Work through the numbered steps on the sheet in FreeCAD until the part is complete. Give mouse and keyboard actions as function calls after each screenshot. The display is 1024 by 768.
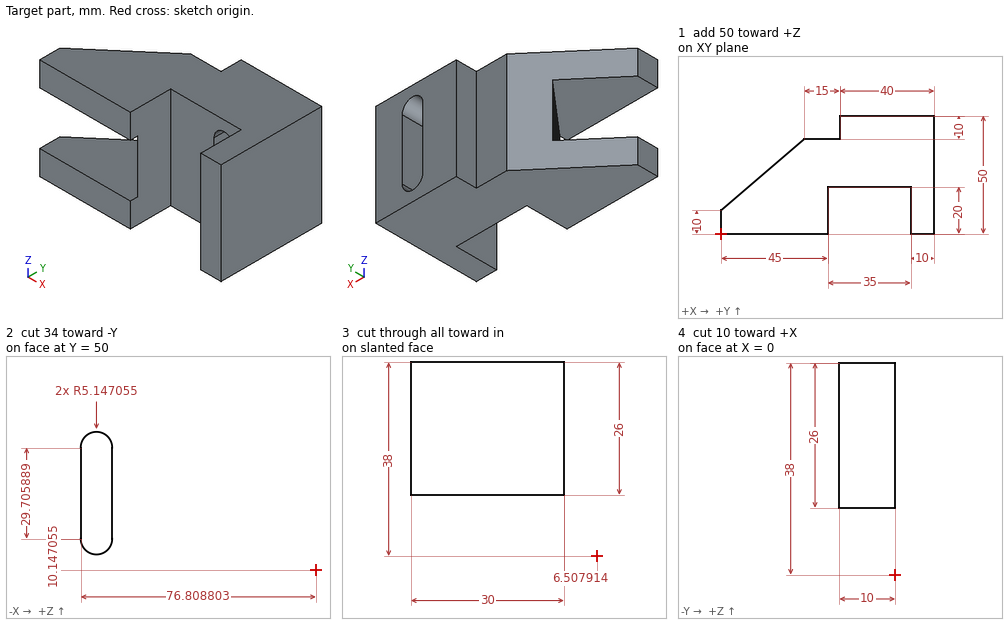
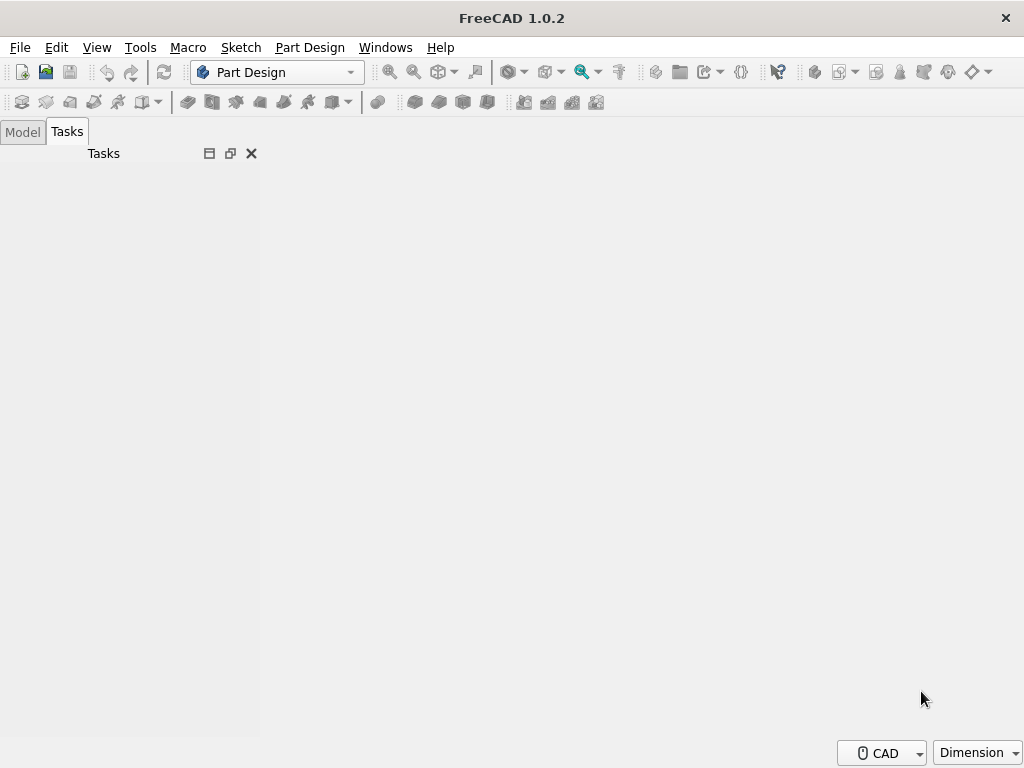
key(ctrl+n)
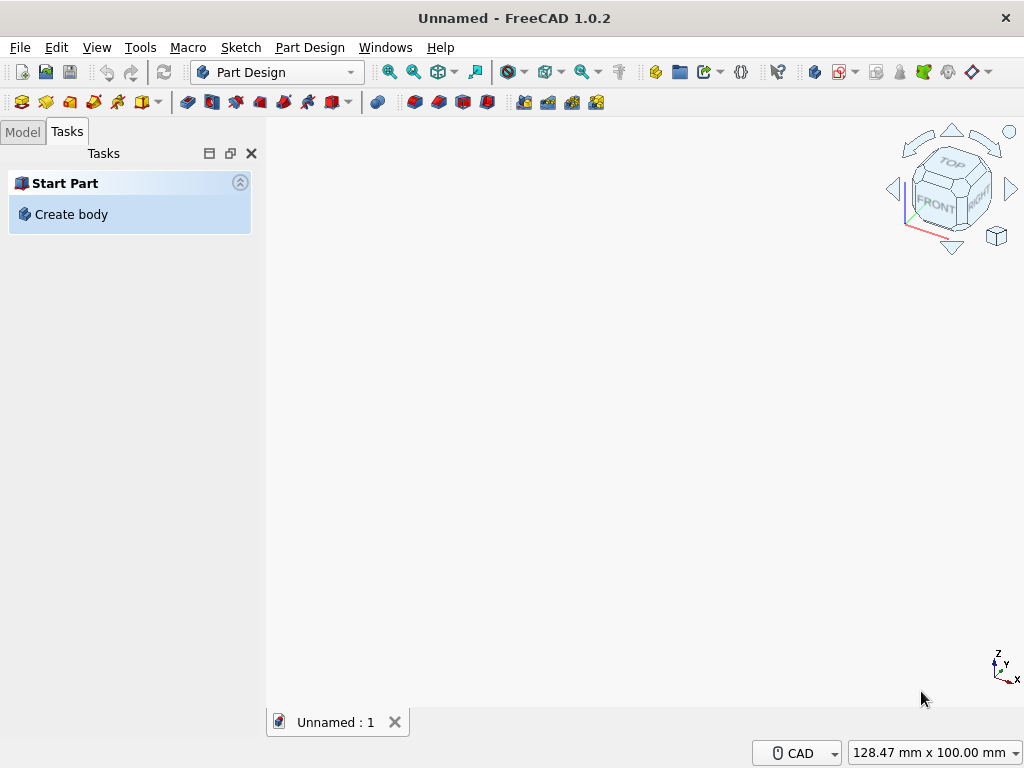
click(840, 72)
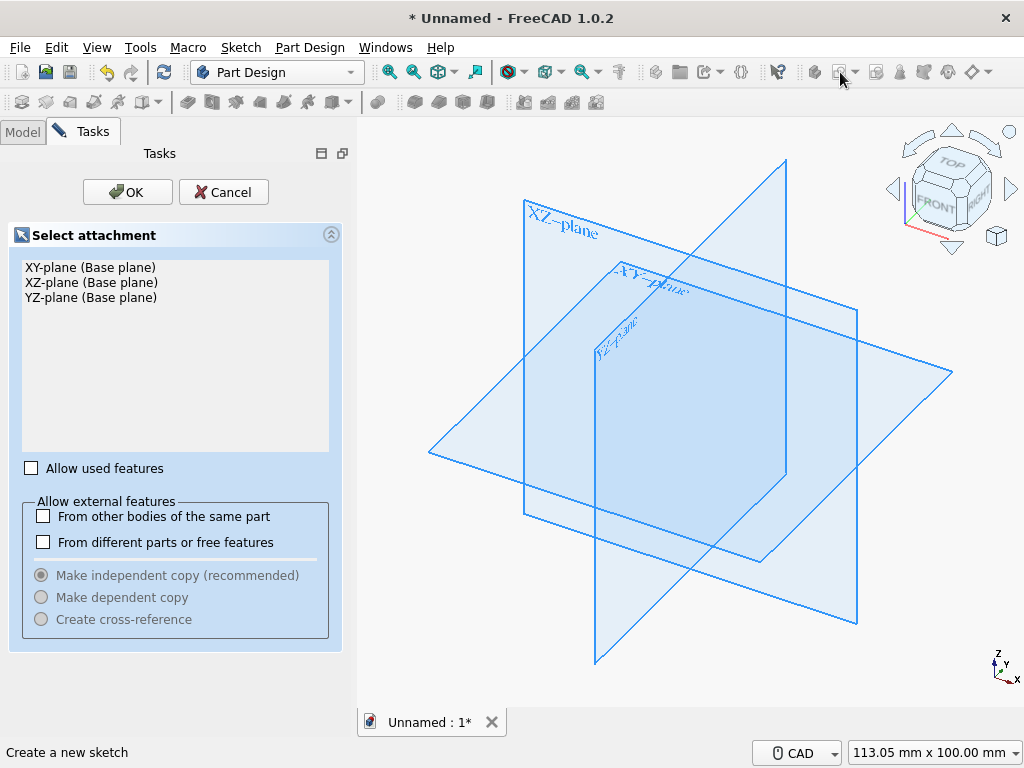
click(82, 268)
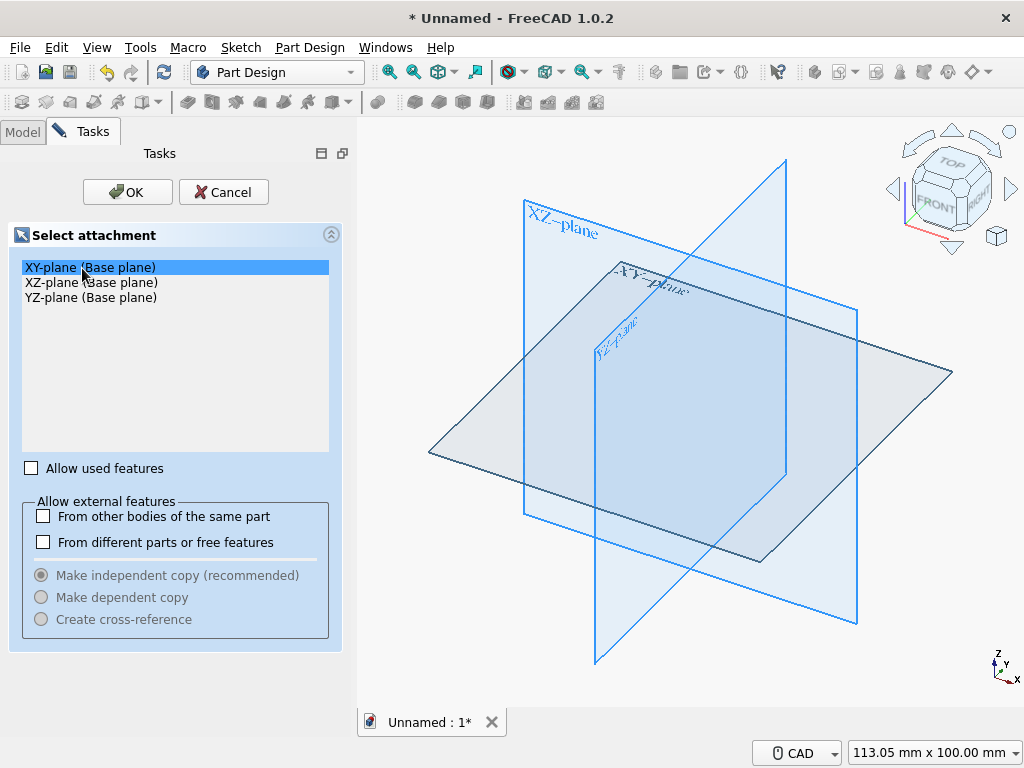
click(128, 192)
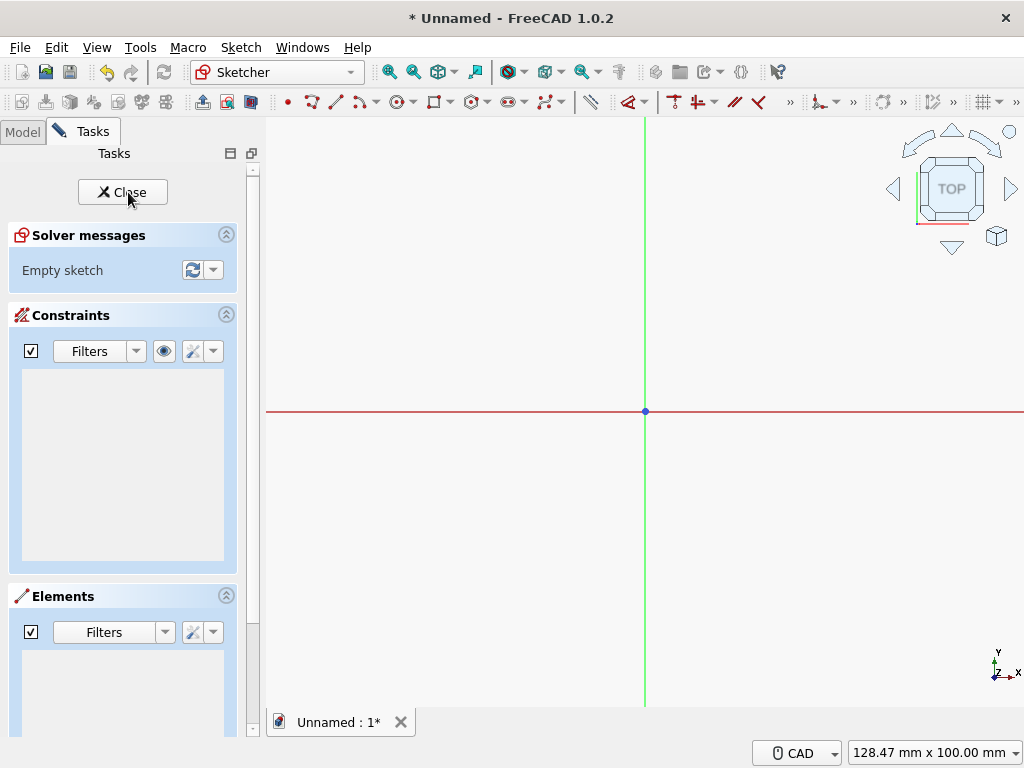
scroll(294, 591, down, 3)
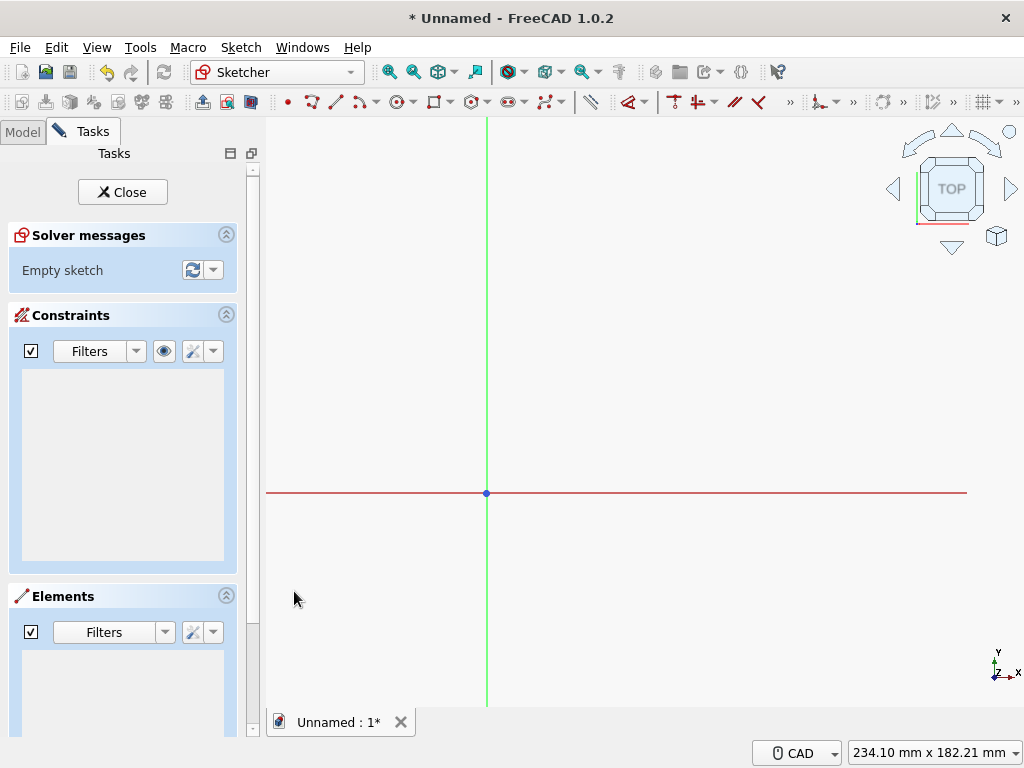
scroll(746, 413, up, 2)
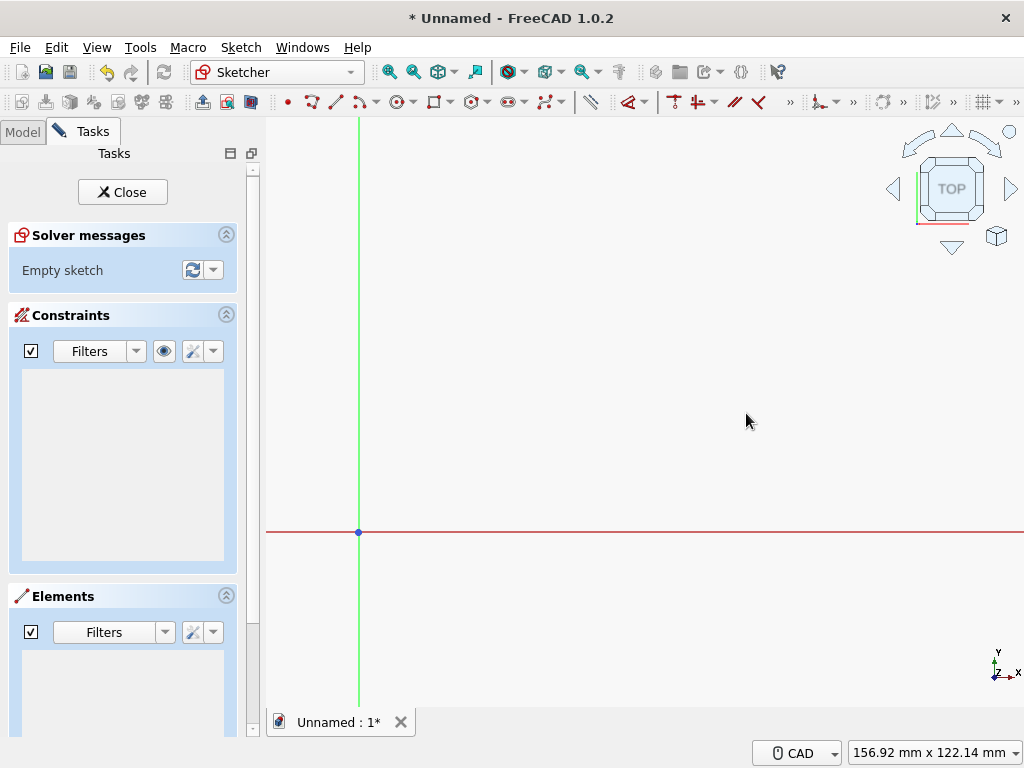
click(312, 102)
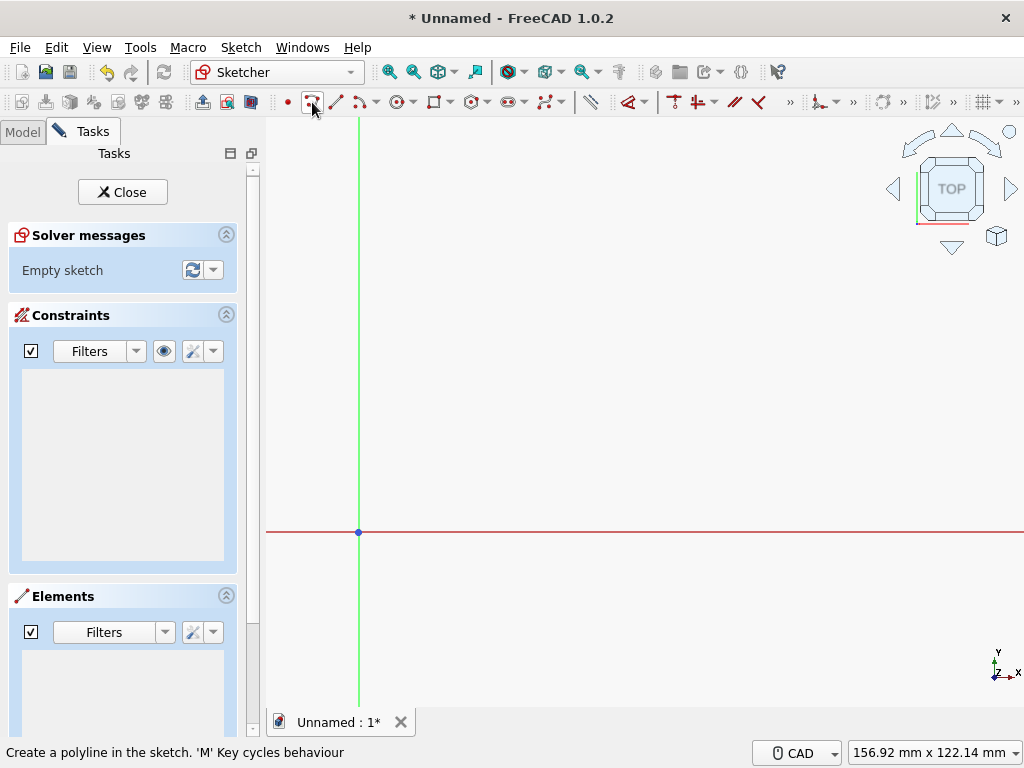
click(359, 532)
click(576, 523)
click(576, 436)
click(745, 436)
click(745, 532)
click(794, 523)
click(794, 291)
click(600, 291)
click(600, 339)
click(528, 339)
click(368, 484)
click(359, 532)
key(Escape)
key(Escape)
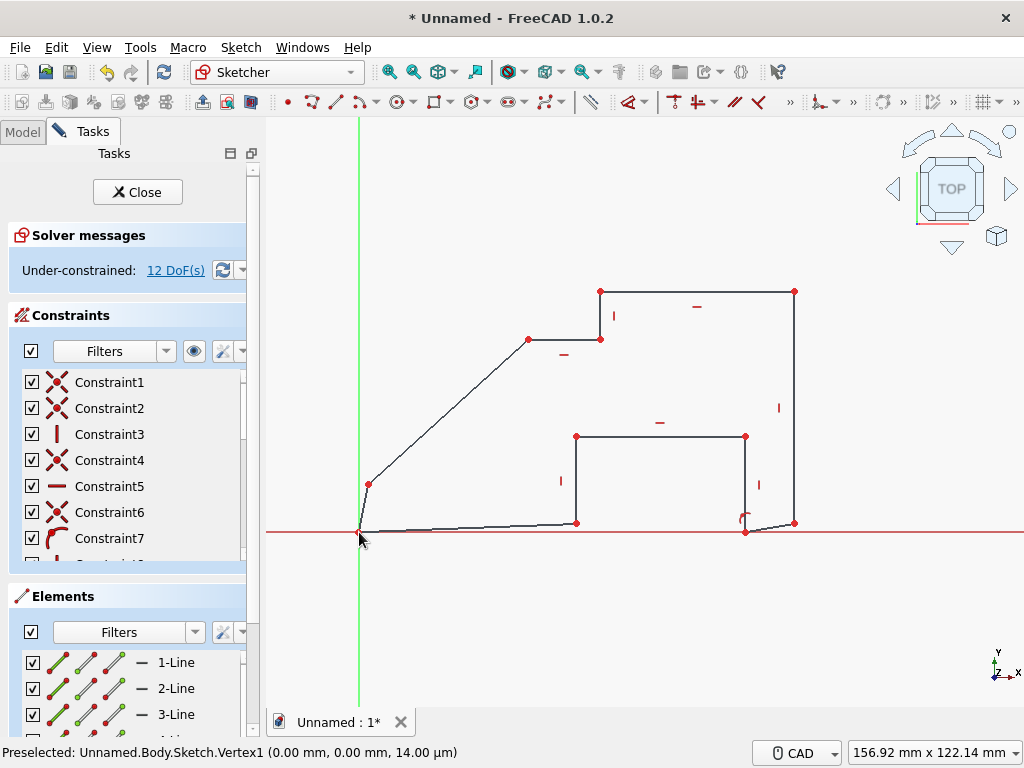
click(424, 530)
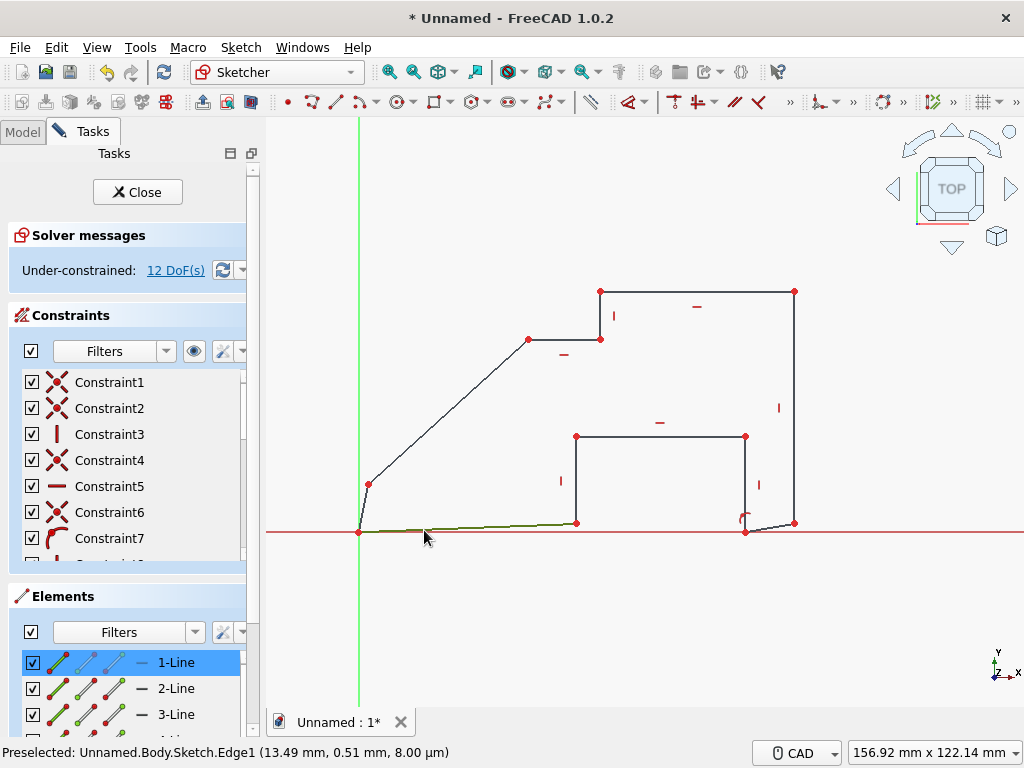
click(716, 102)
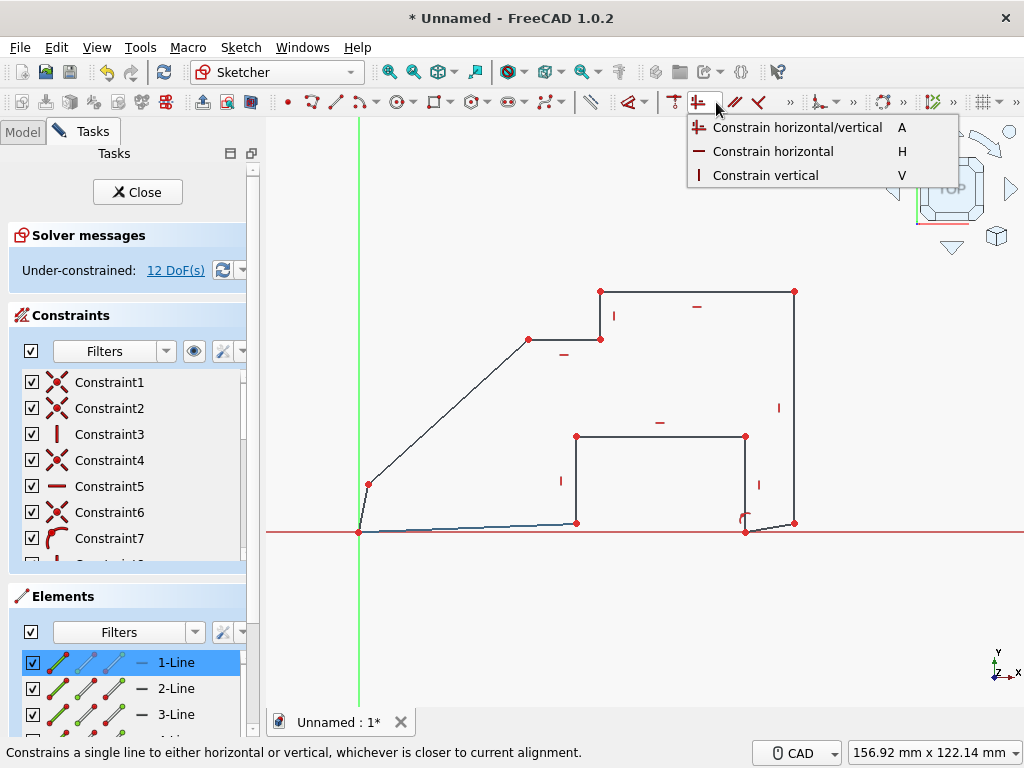
click(823, 151)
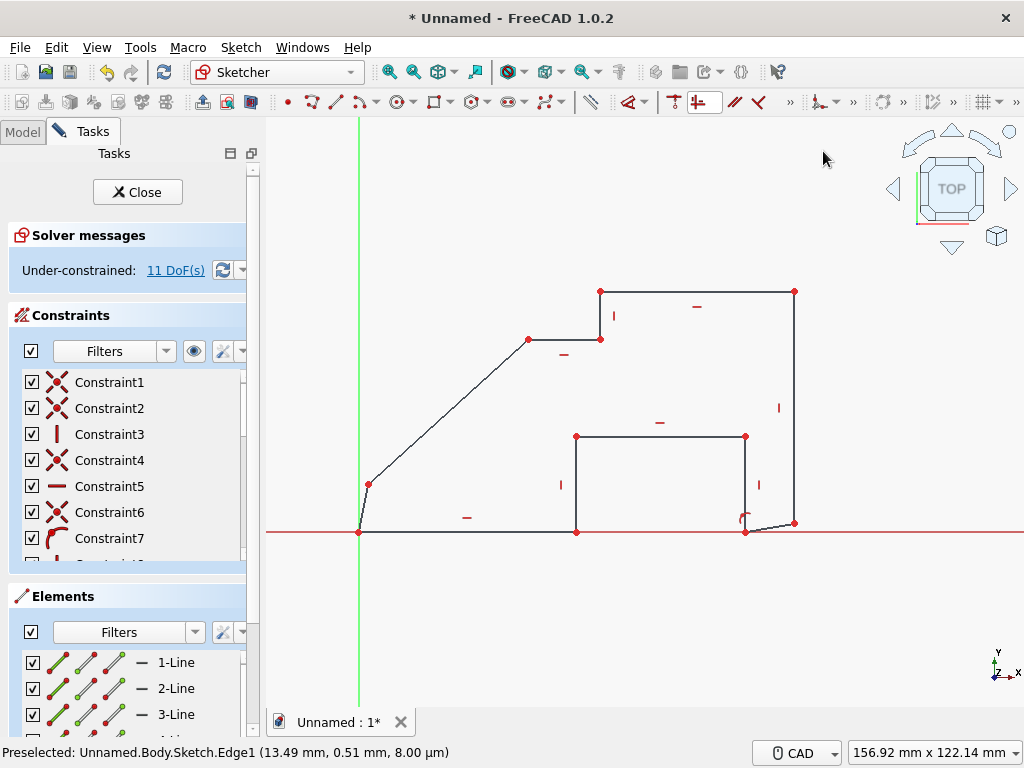
click(760, 530)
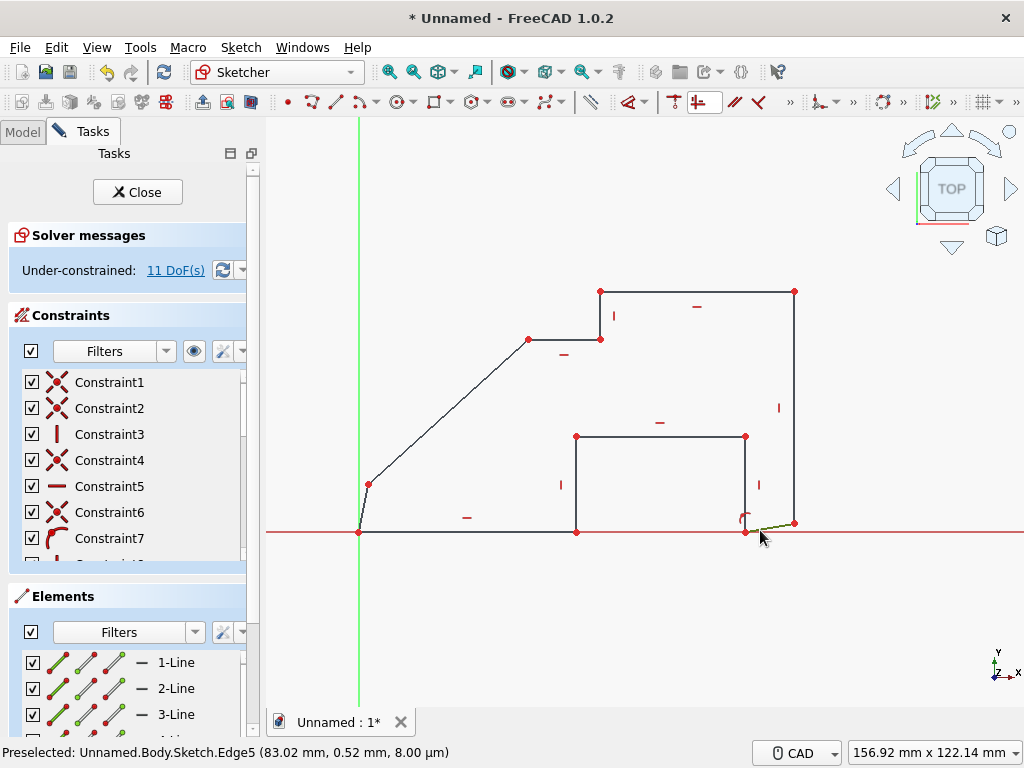
click(716, 102)